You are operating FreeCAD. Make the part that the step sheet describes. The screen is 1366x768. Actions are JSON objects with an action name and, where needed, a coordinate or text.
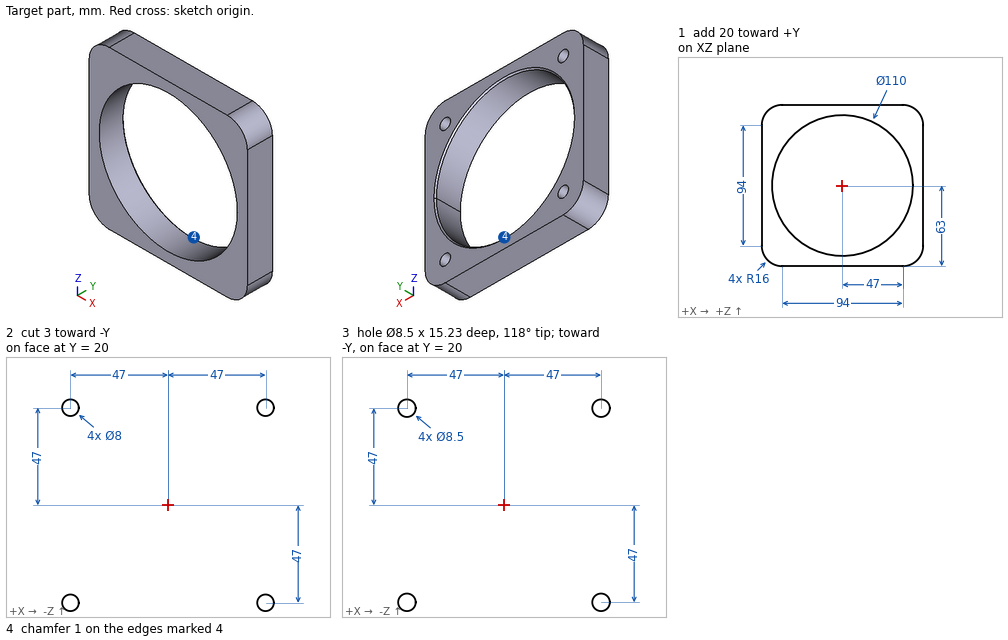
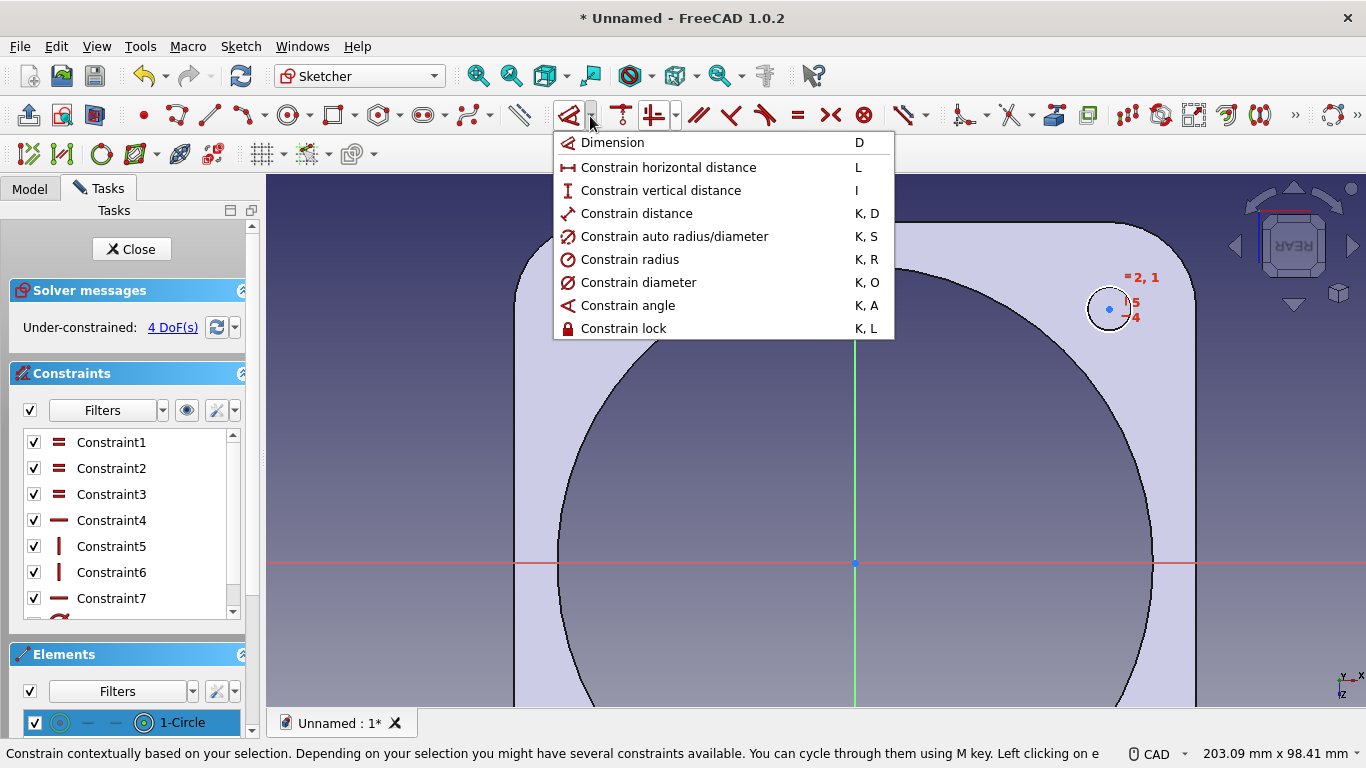
{"action": "left_click", "coordinate": [724, 168]}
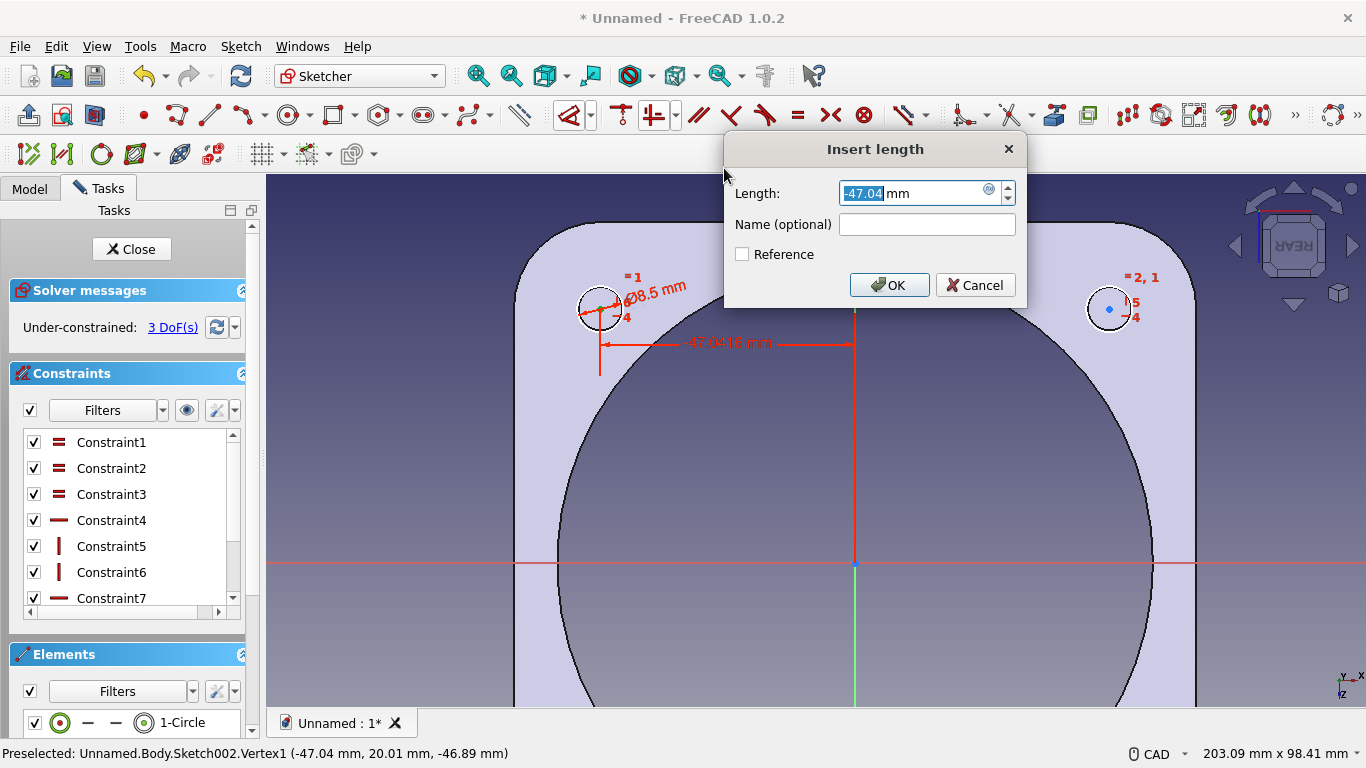
{"action": "type", "text": "-47"}
{"action": "key", "text": "Return"}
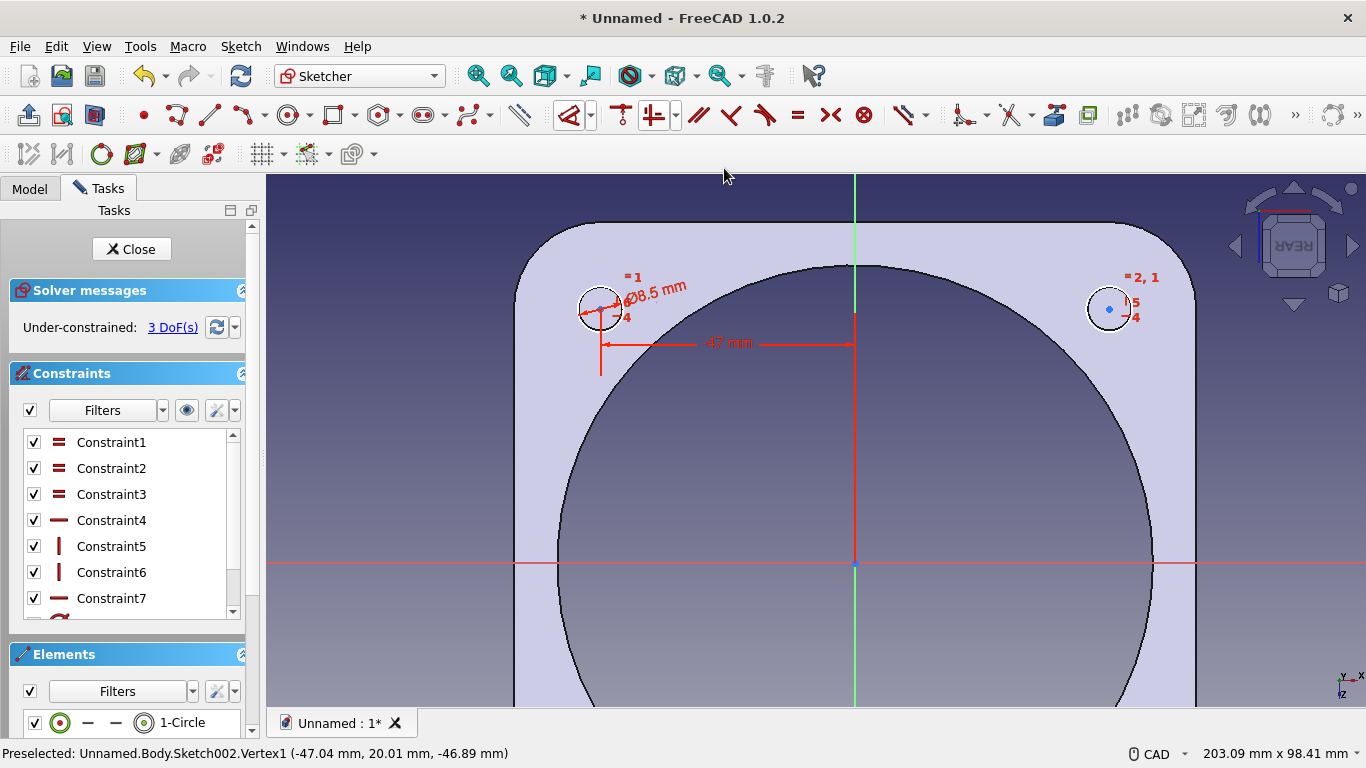
{"action": "left_click", "coordinate": [601, 309]}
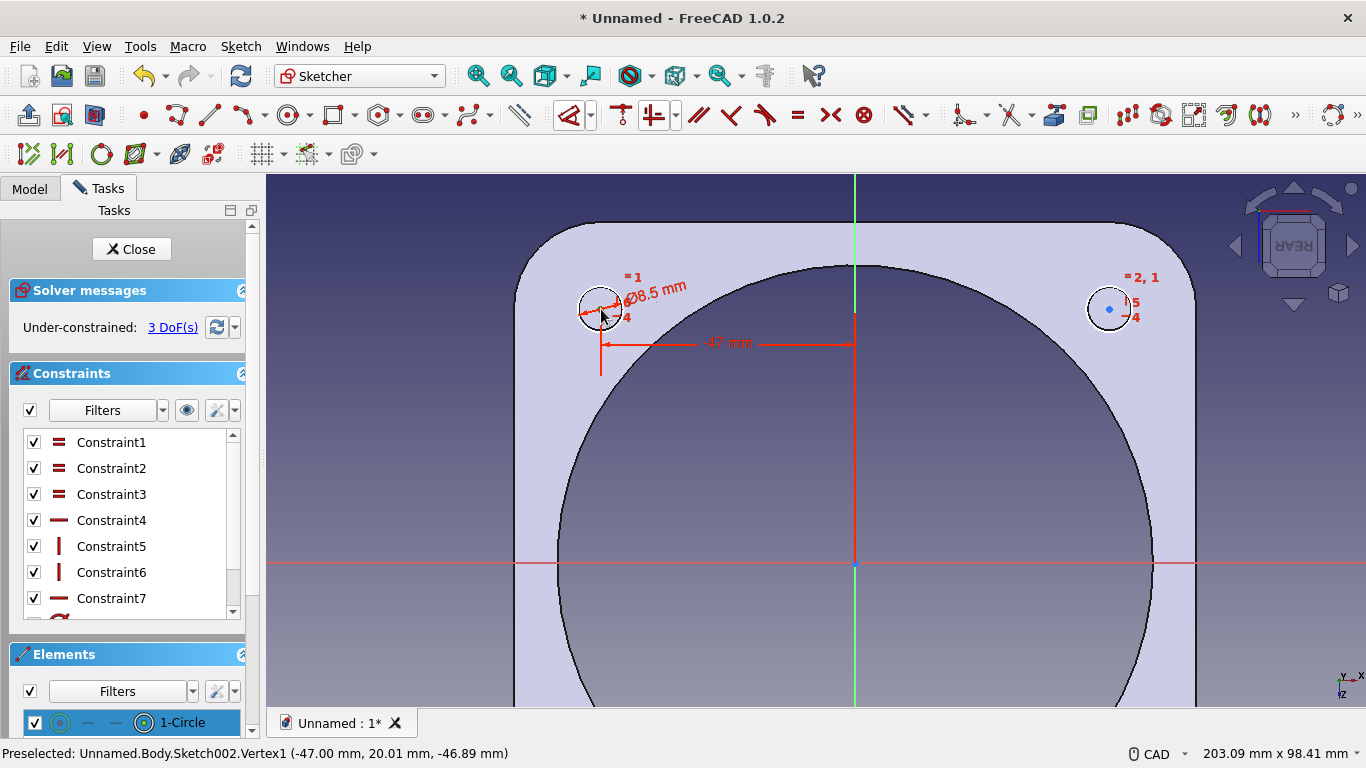
{"action": "left_click", "coordinate": [590, 116]}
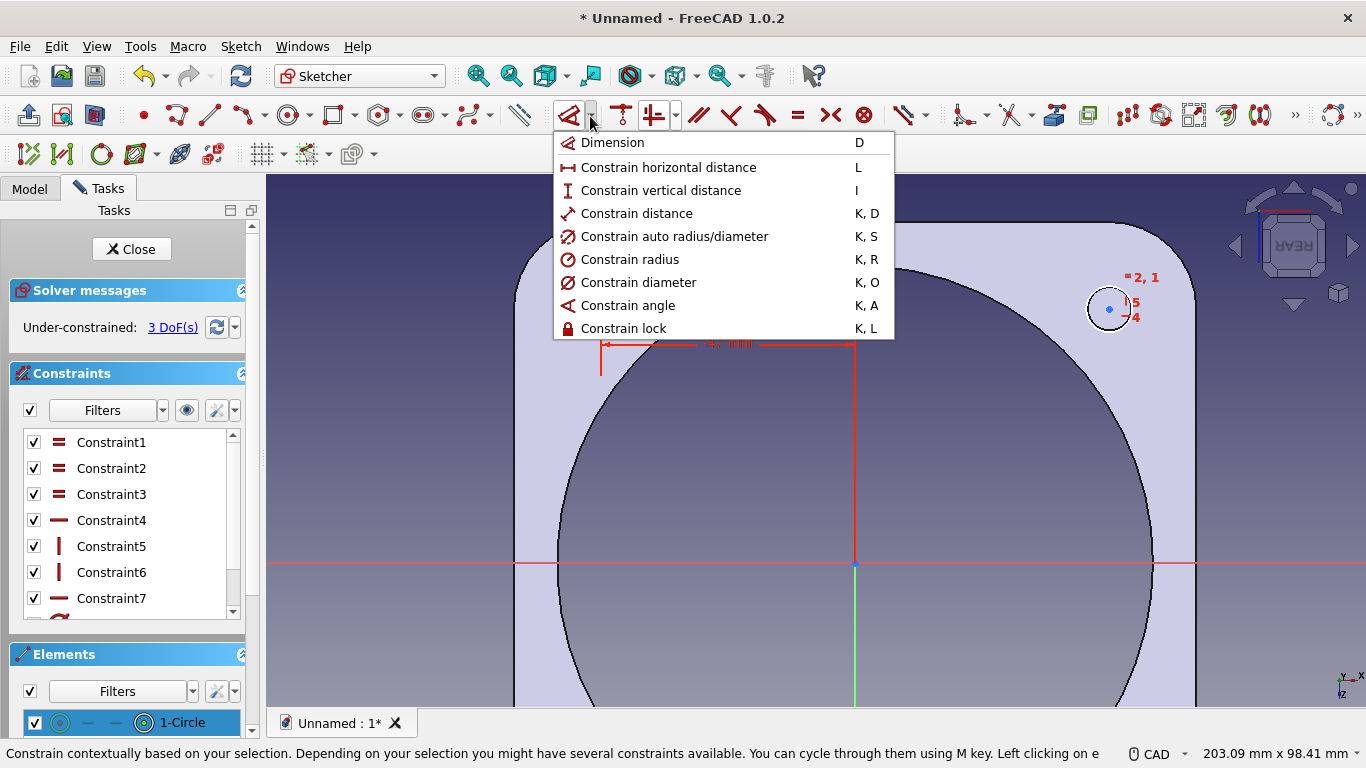
{"action": "left_click", "coordinate": [724, 190]}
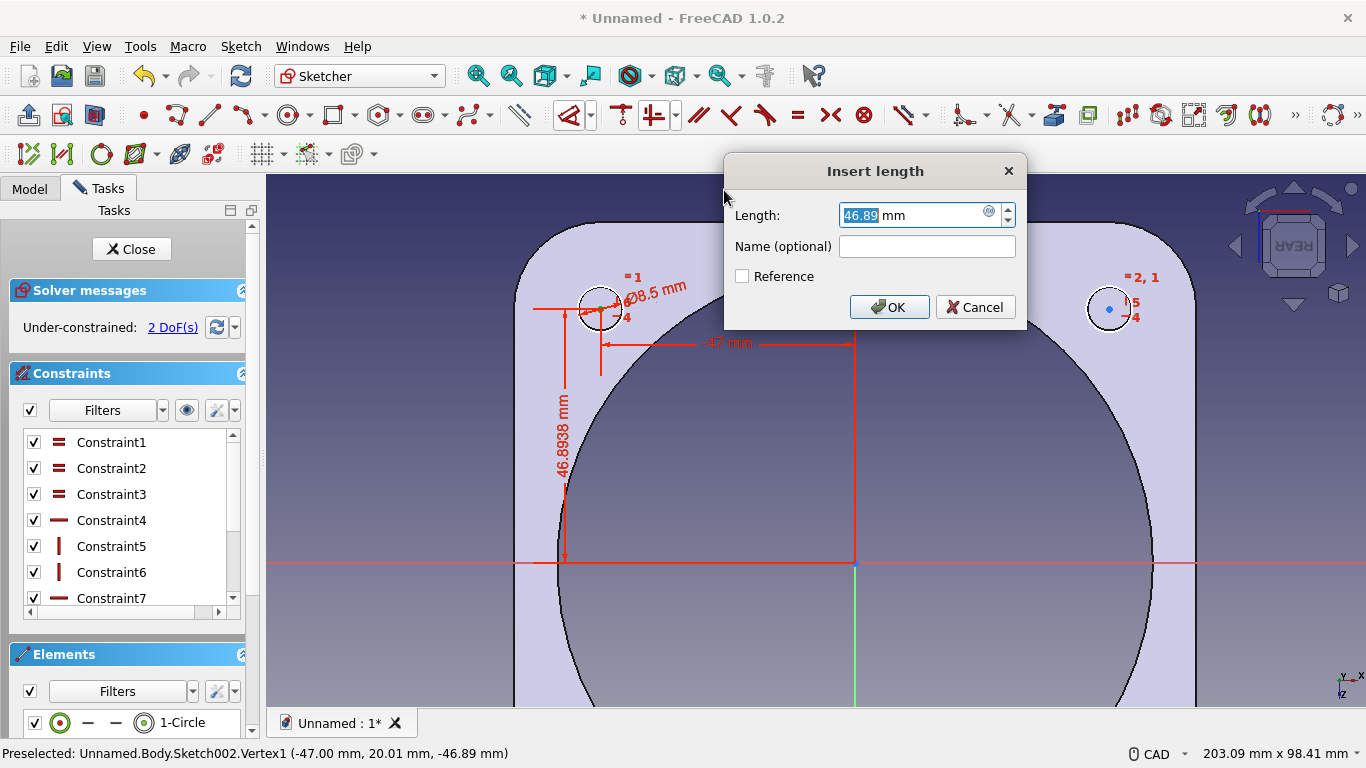
{"action": "type", "text": "47"}
{"action": "key", "text": "Return"}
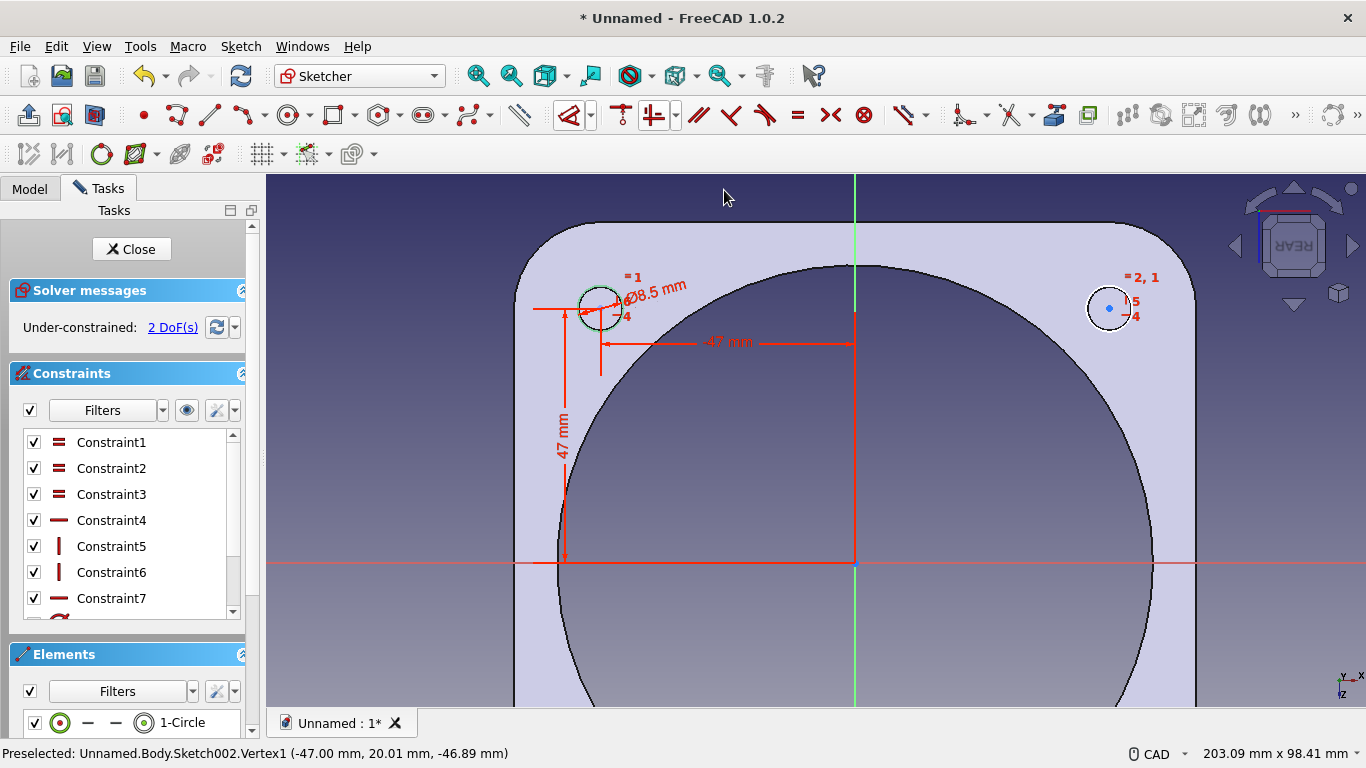
{"action": "left_click", "coordinate": [1109, 309]}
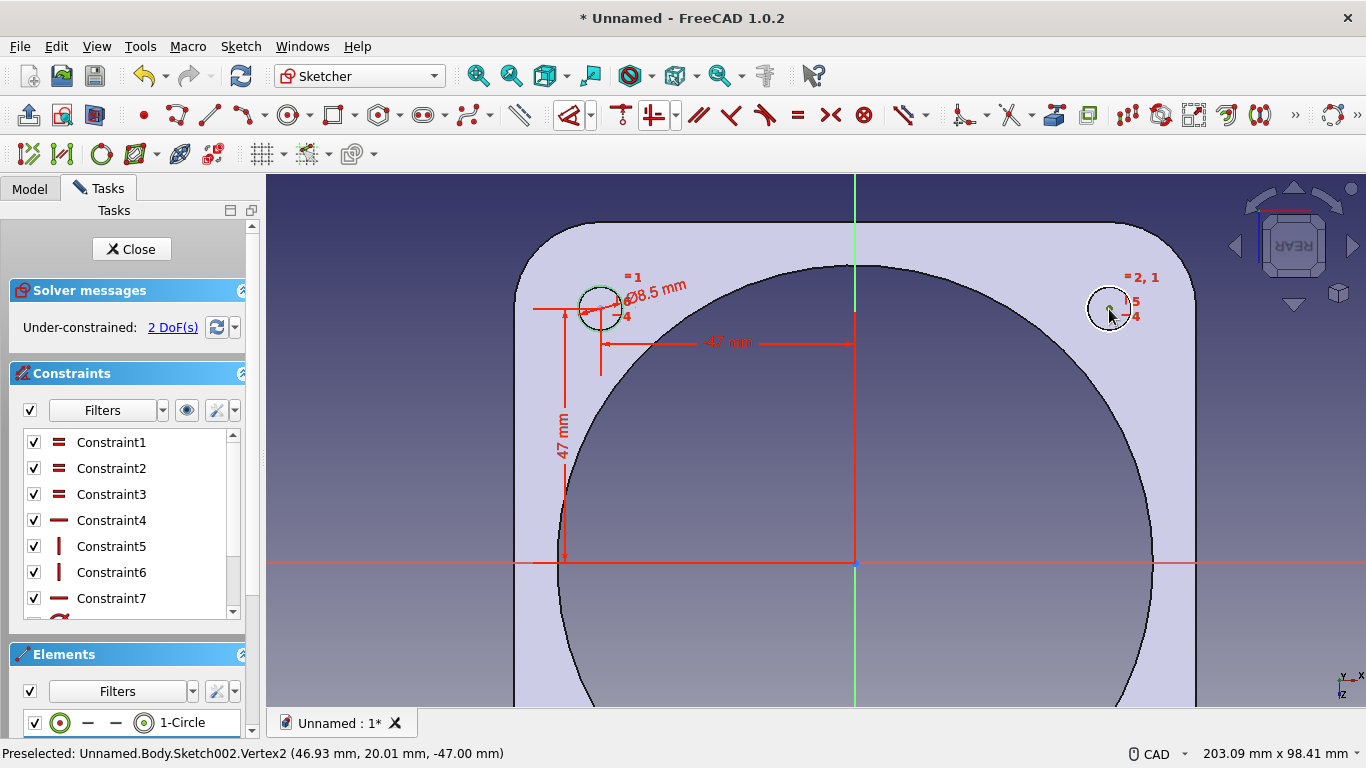
{"action": "left_click", "coordinate": [590, 116]}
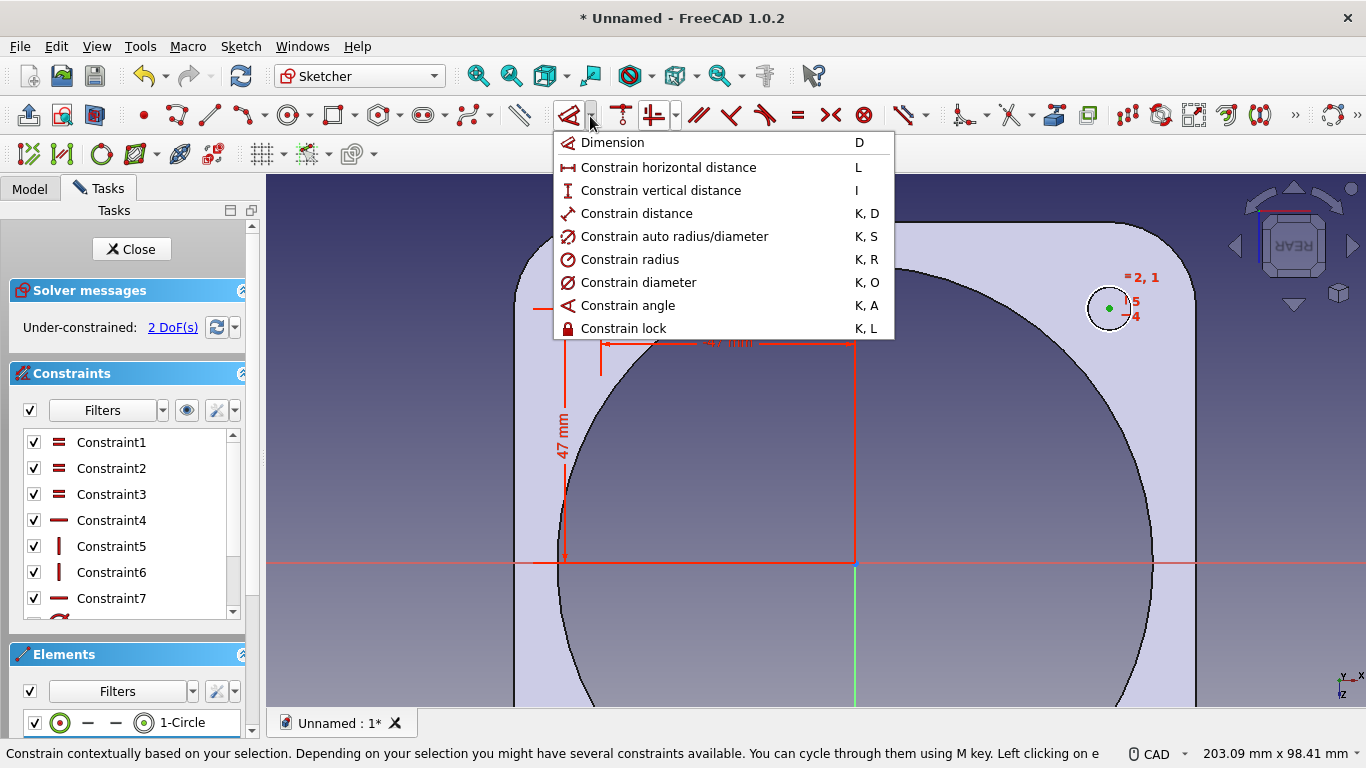
{"action": "left_click", "coordinate": [724, 168]}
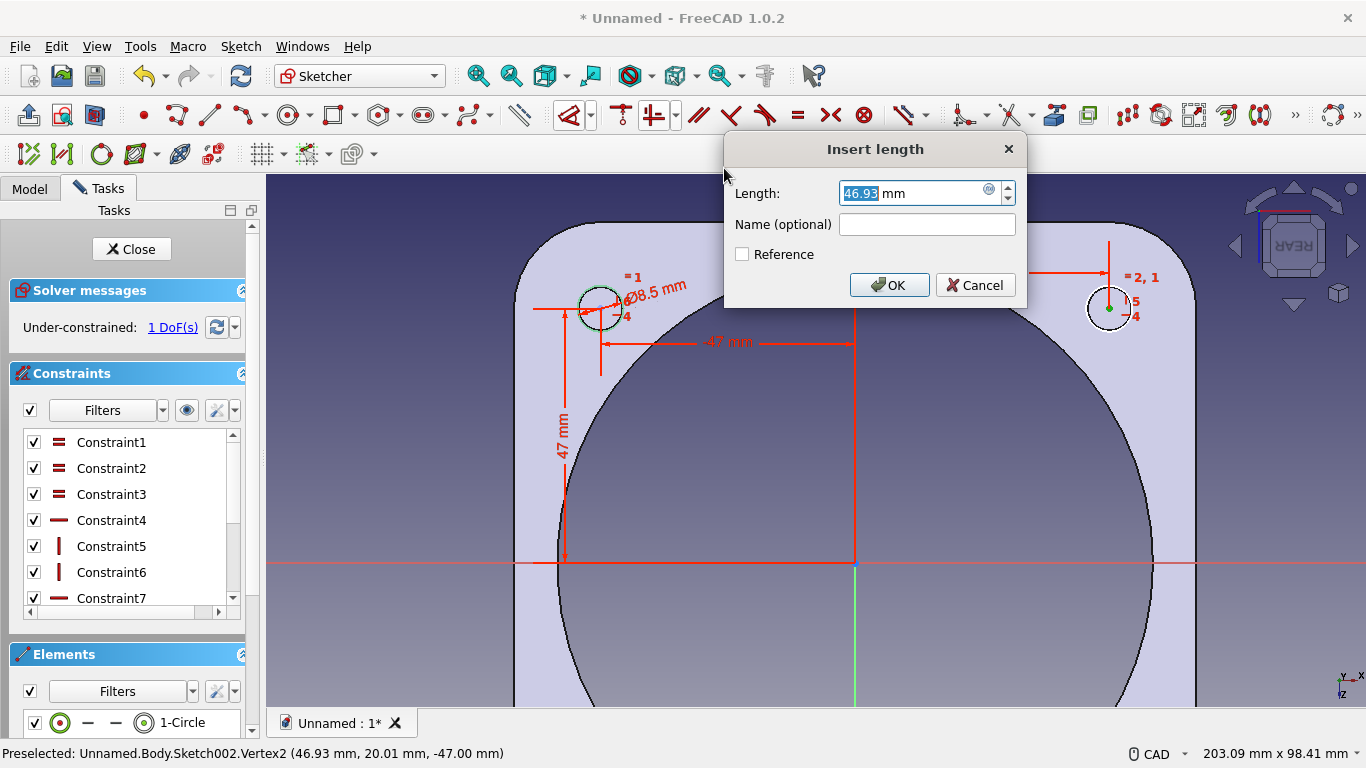
{"action": "type", "text": "47"}
{"action": "key", "text": "Return"}